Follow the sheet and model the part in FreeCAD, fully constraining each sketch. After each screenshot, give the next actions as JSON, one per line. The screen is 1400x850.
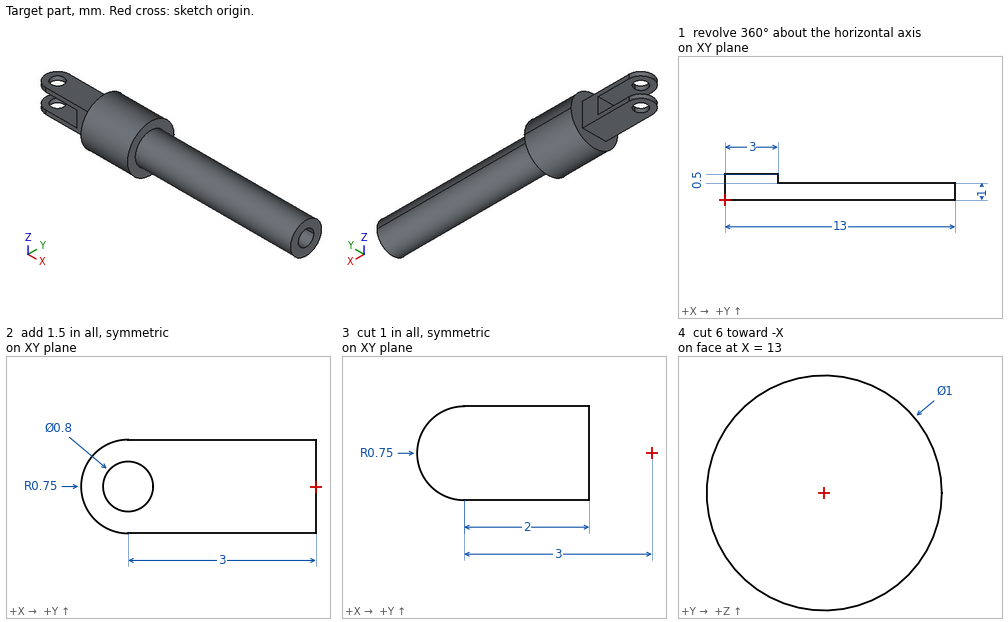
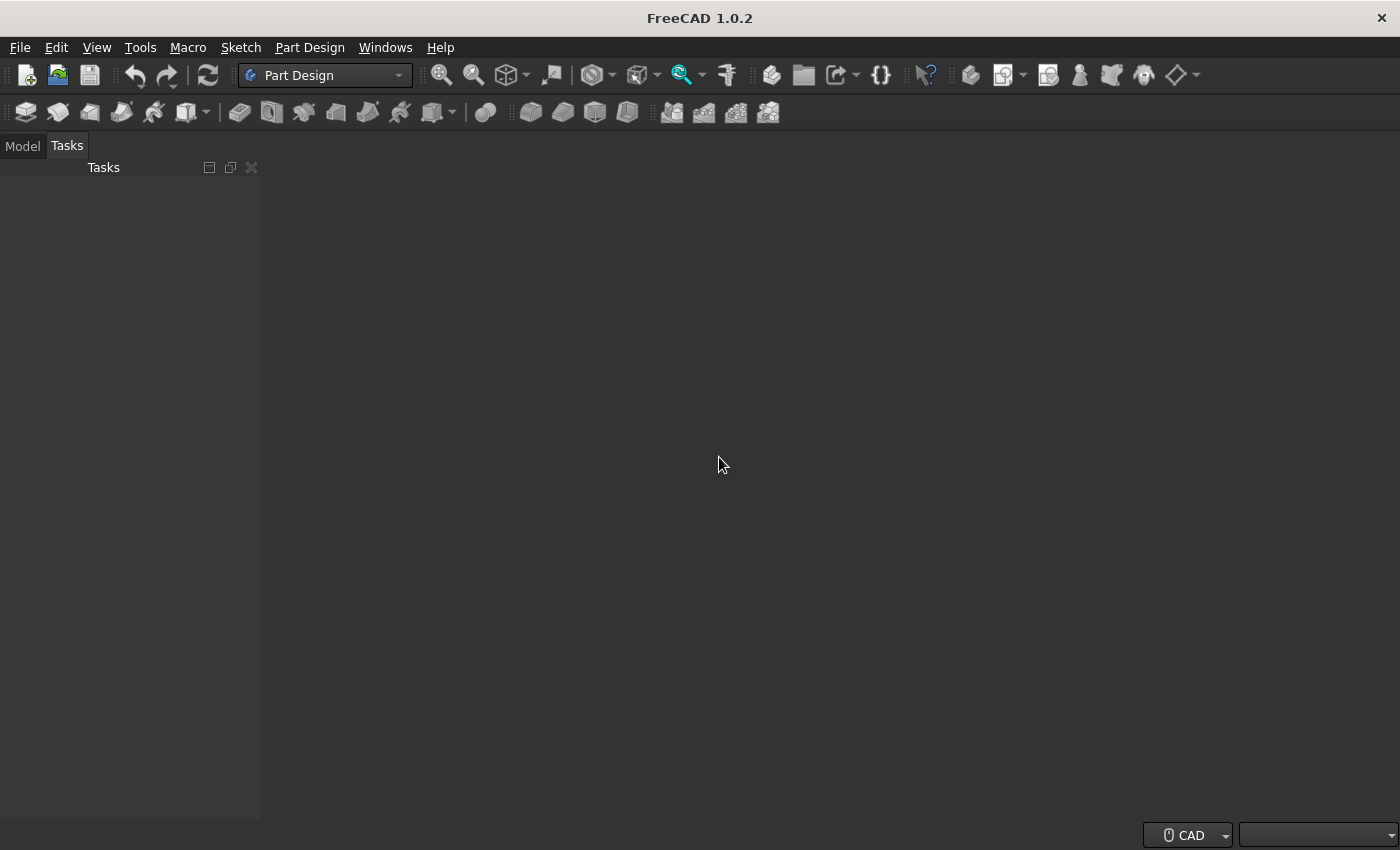
{"action": "left_click", "coordinate": [26, 76]}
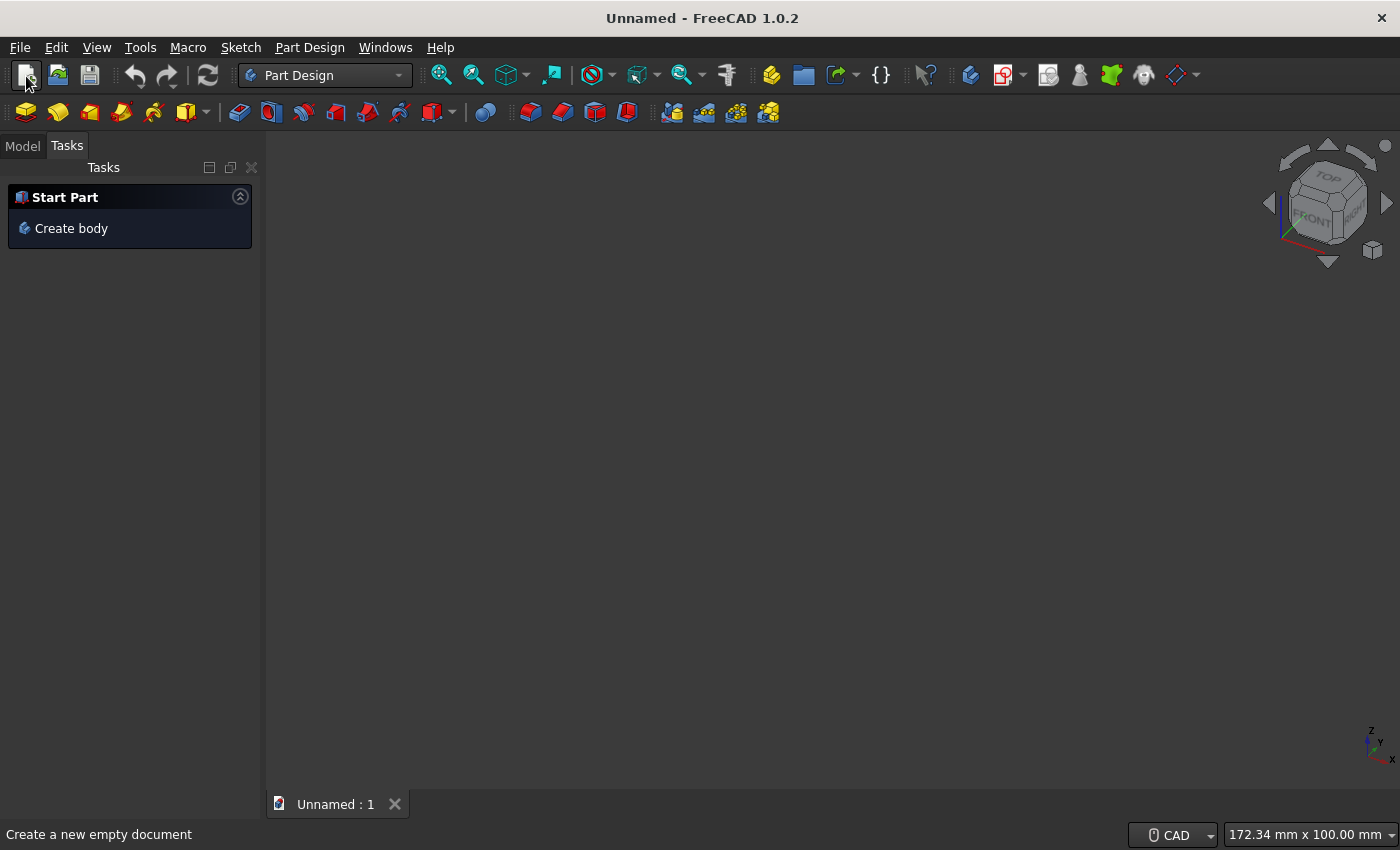
{"action": "left_click", "coordinate": [1004, 76]}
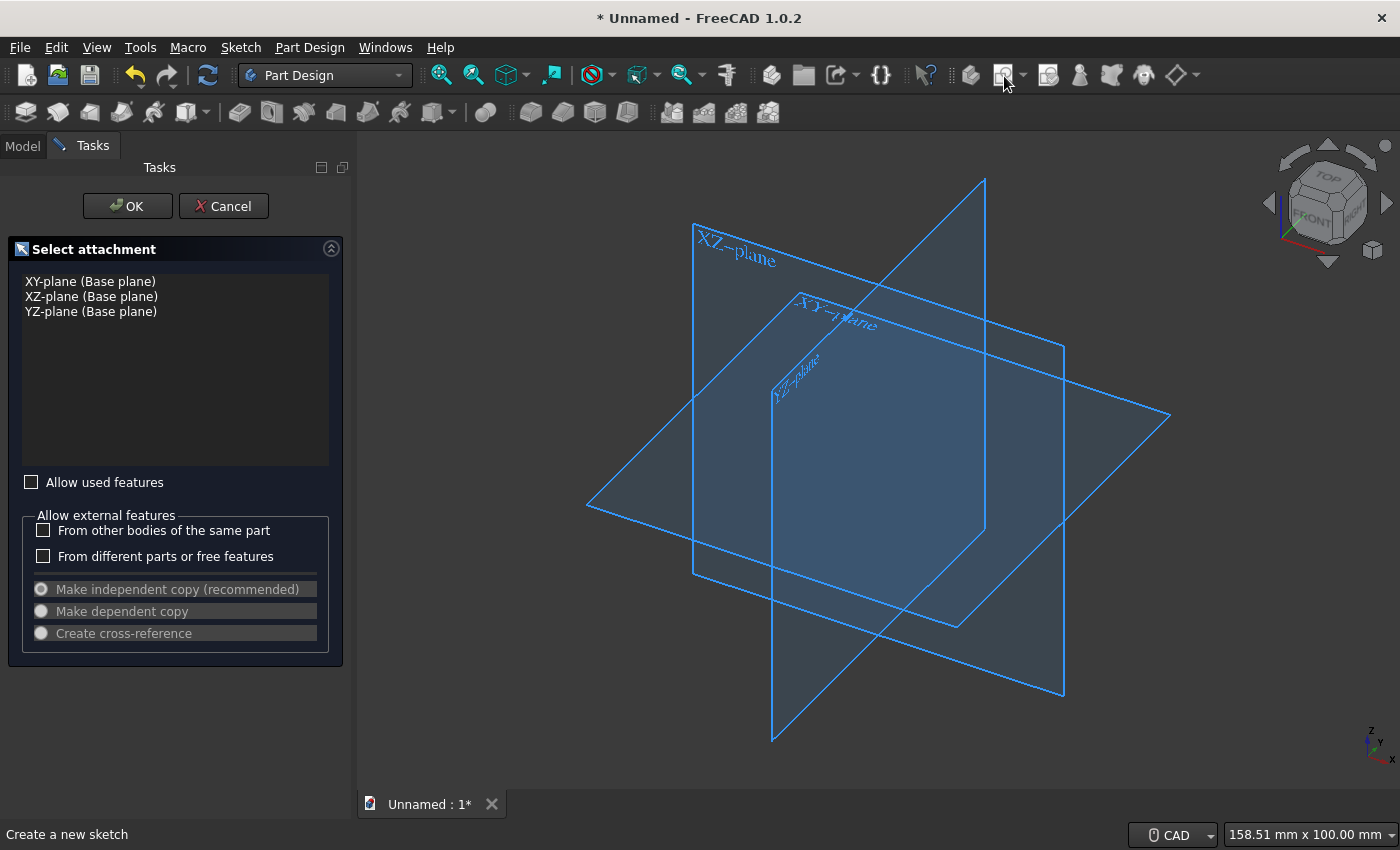
{"action": "left_click", "coordinate": [82, 282]}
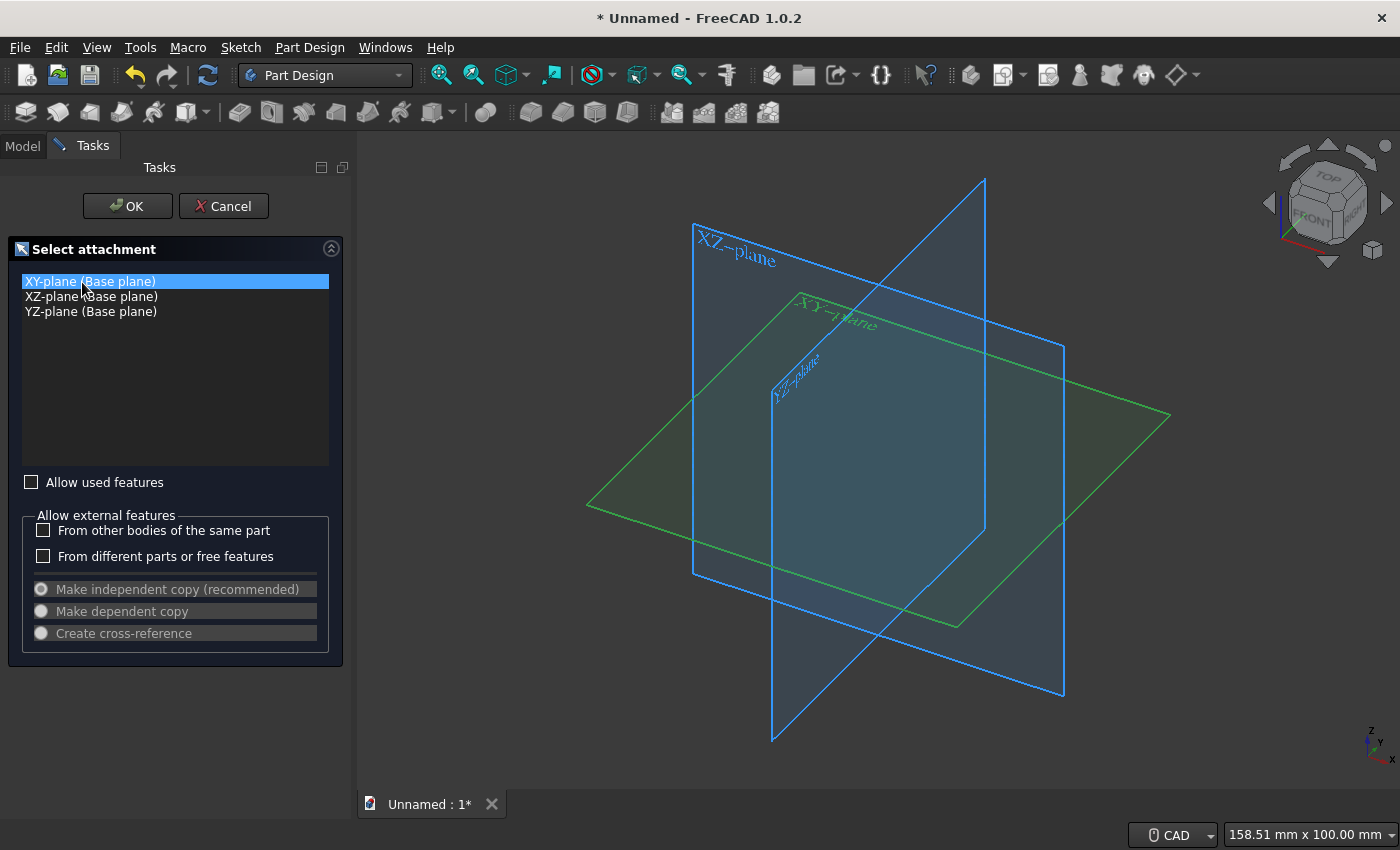
{"action": "left_click", "coordinate": [128, 206]}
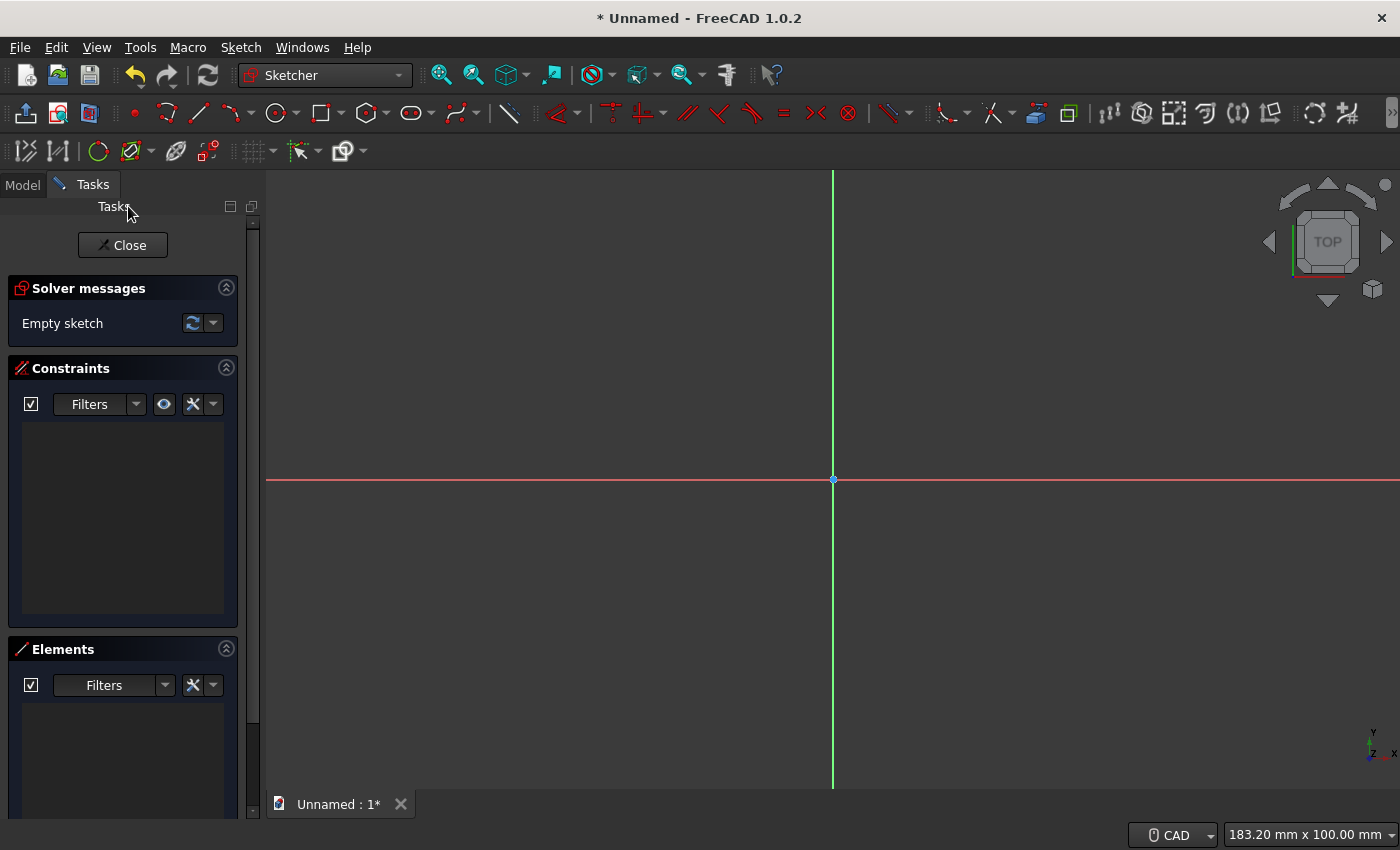
{"action": "scroll", "coordinate": [887, 474], "scroll_direction": "up", "scroll_amount": 11}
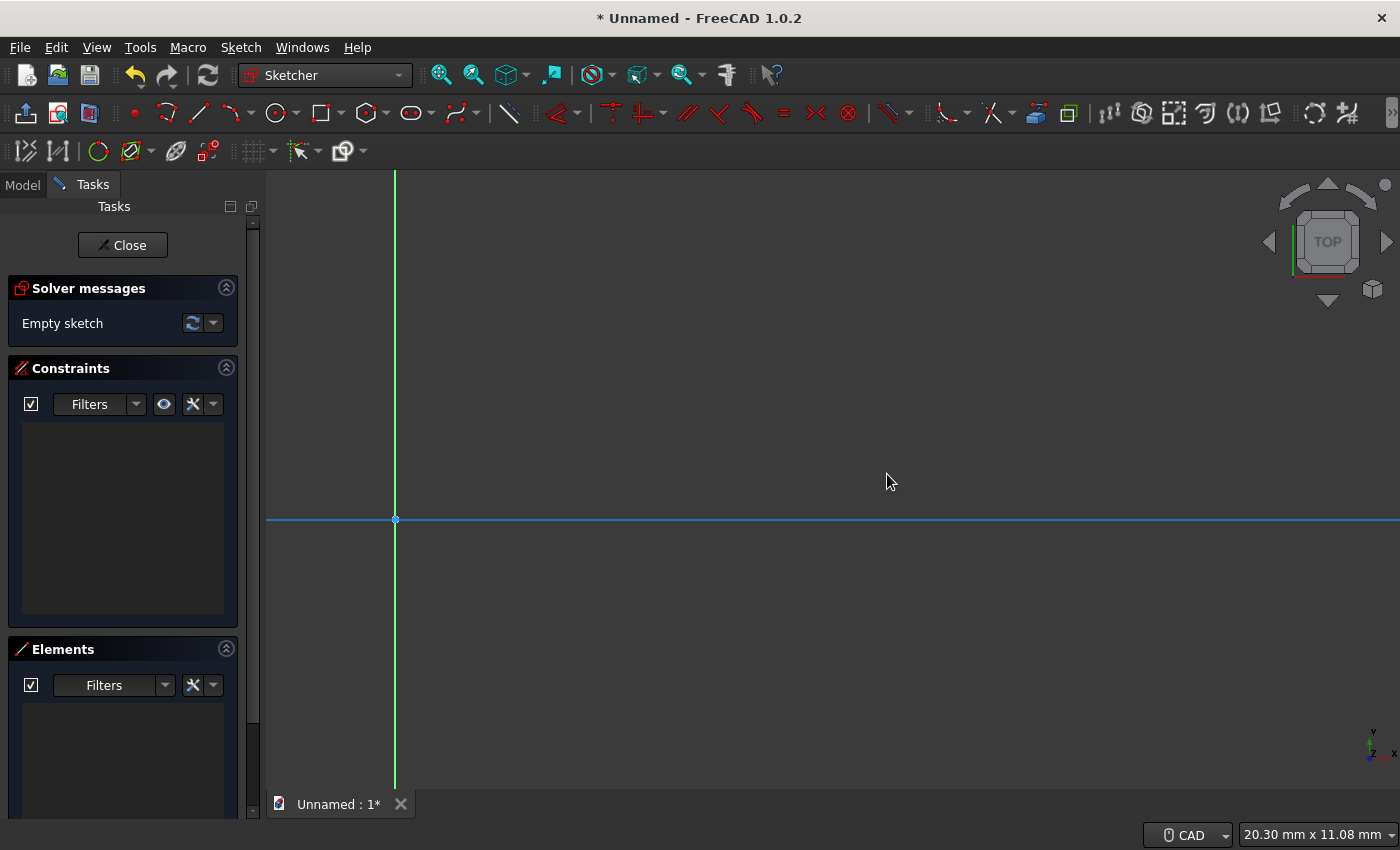
{"action": "left_click", "coordinate": [168, 114]}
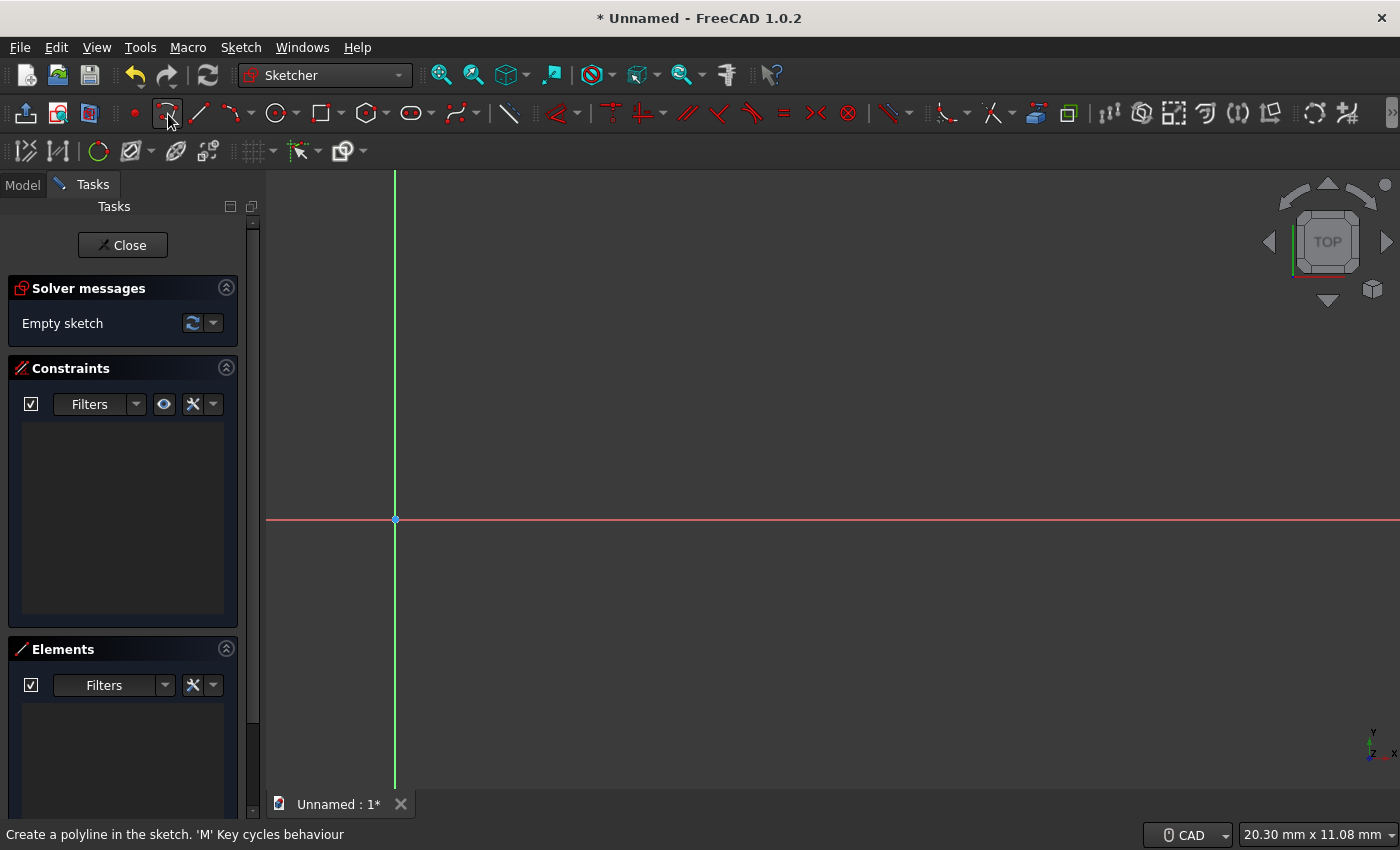
{"action": "left_click", "coordinate": [395, 520]}
{"action": "left_click", "coordinate": [1121, 511]}
{"action": "left_click", "coordinate": [1121, 464]}
{"action": "left_click", "coordinate": [563, 464]}
{"action": "left_click", "coordinate": [563, 436]}
{"action": "left_click", "coordinate": [404, 436]}
{"action": "left_click", "coordinate": [395, 520]}
{"action": "key", "text": "Escape"}
{"action": "key", "text": "Escape"}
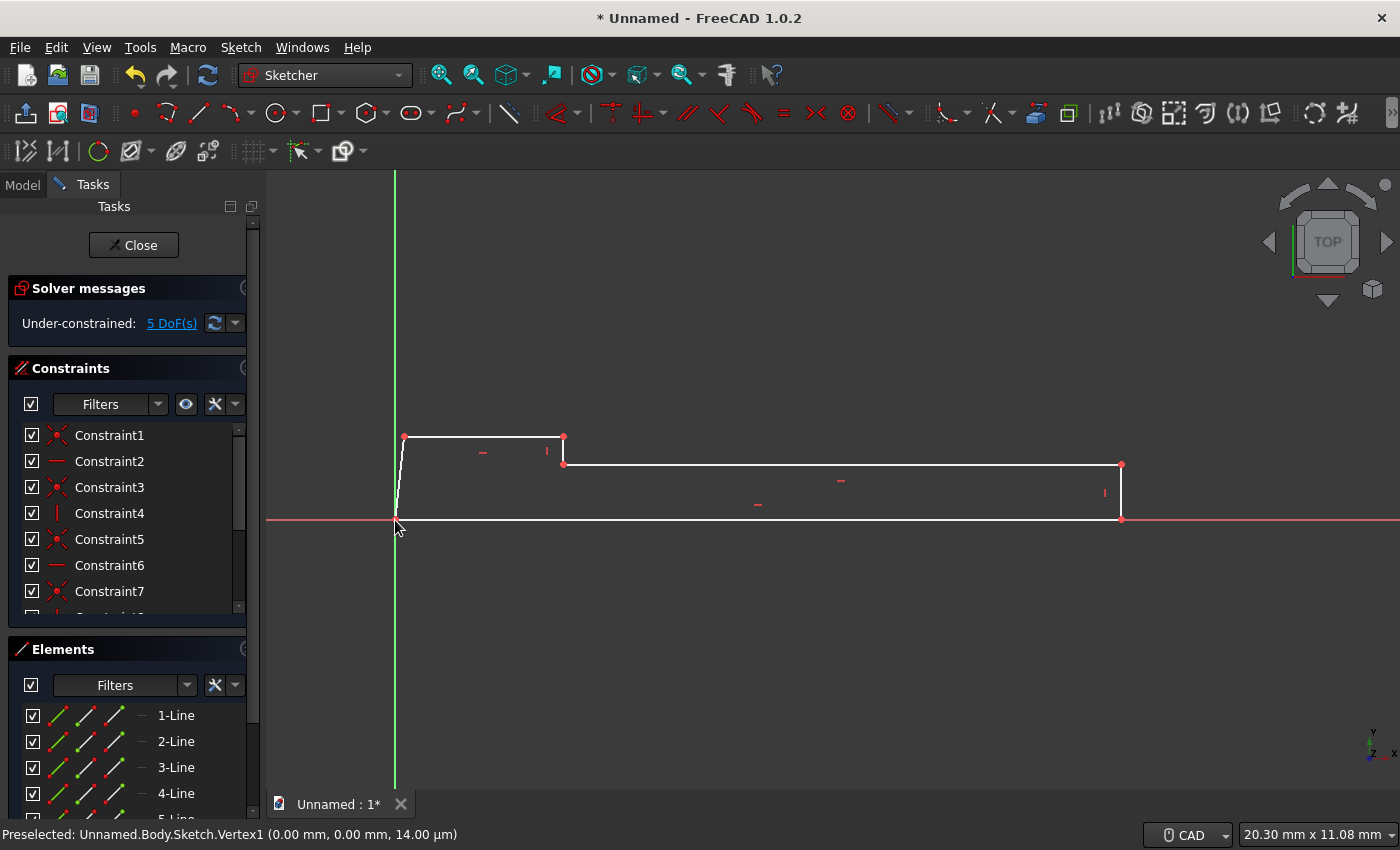
{"action": "left_click", "coordinate": [398, 495]}